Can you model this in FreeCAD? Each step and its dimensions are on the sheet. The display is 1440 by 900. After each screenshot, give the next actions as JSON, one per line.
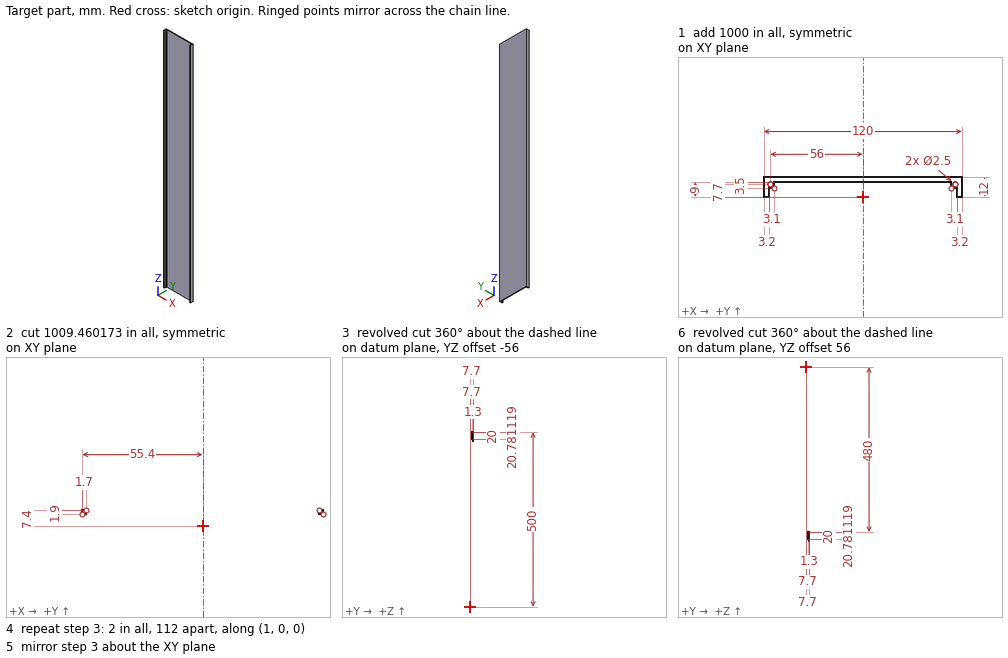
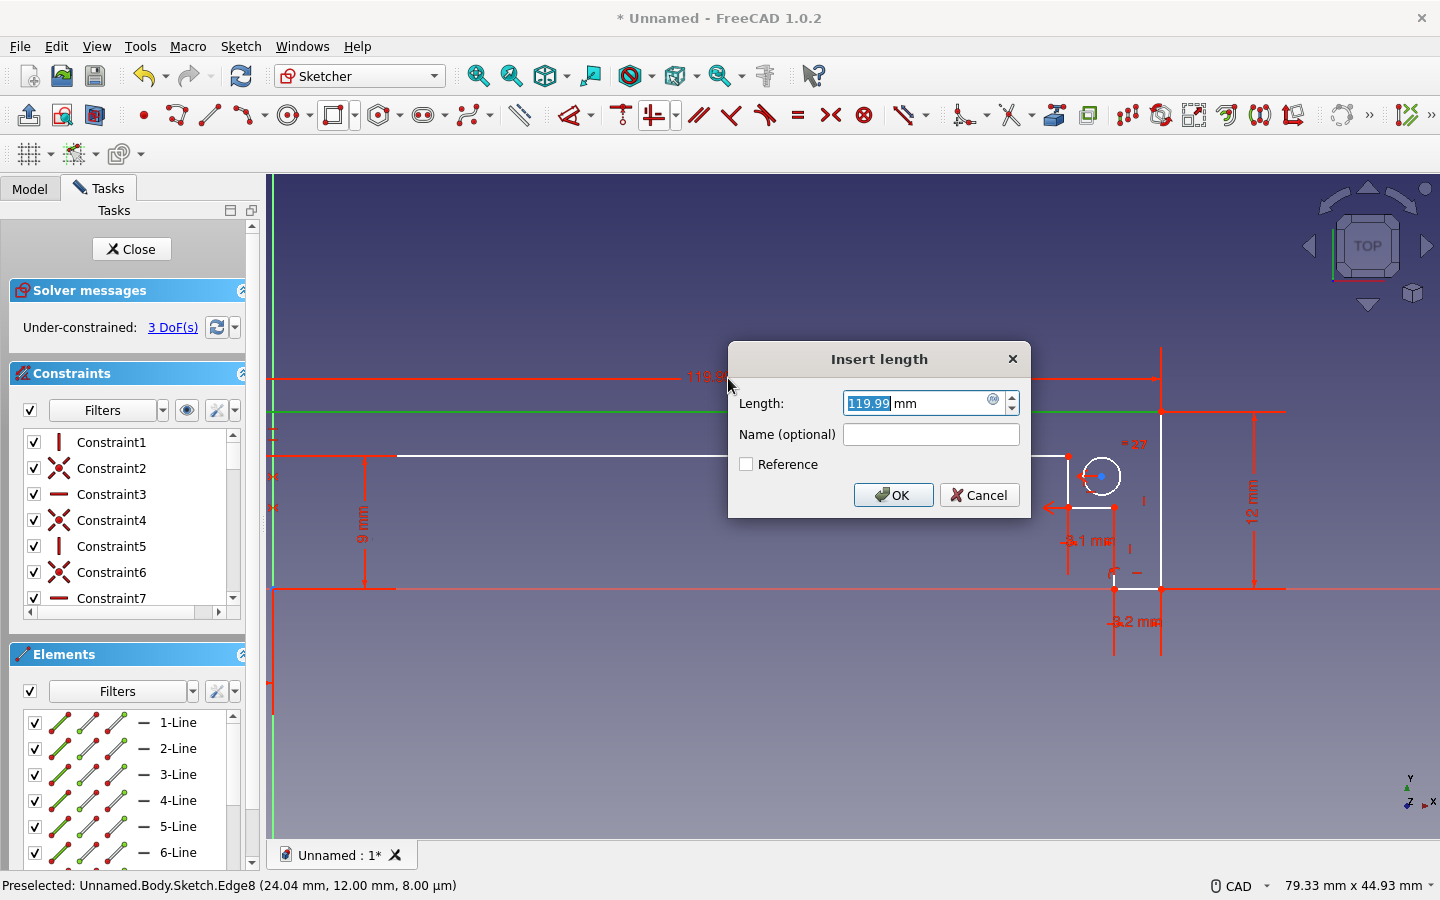
{"action": "type", "text": "120"}
{"action": "key", "text": "Return"}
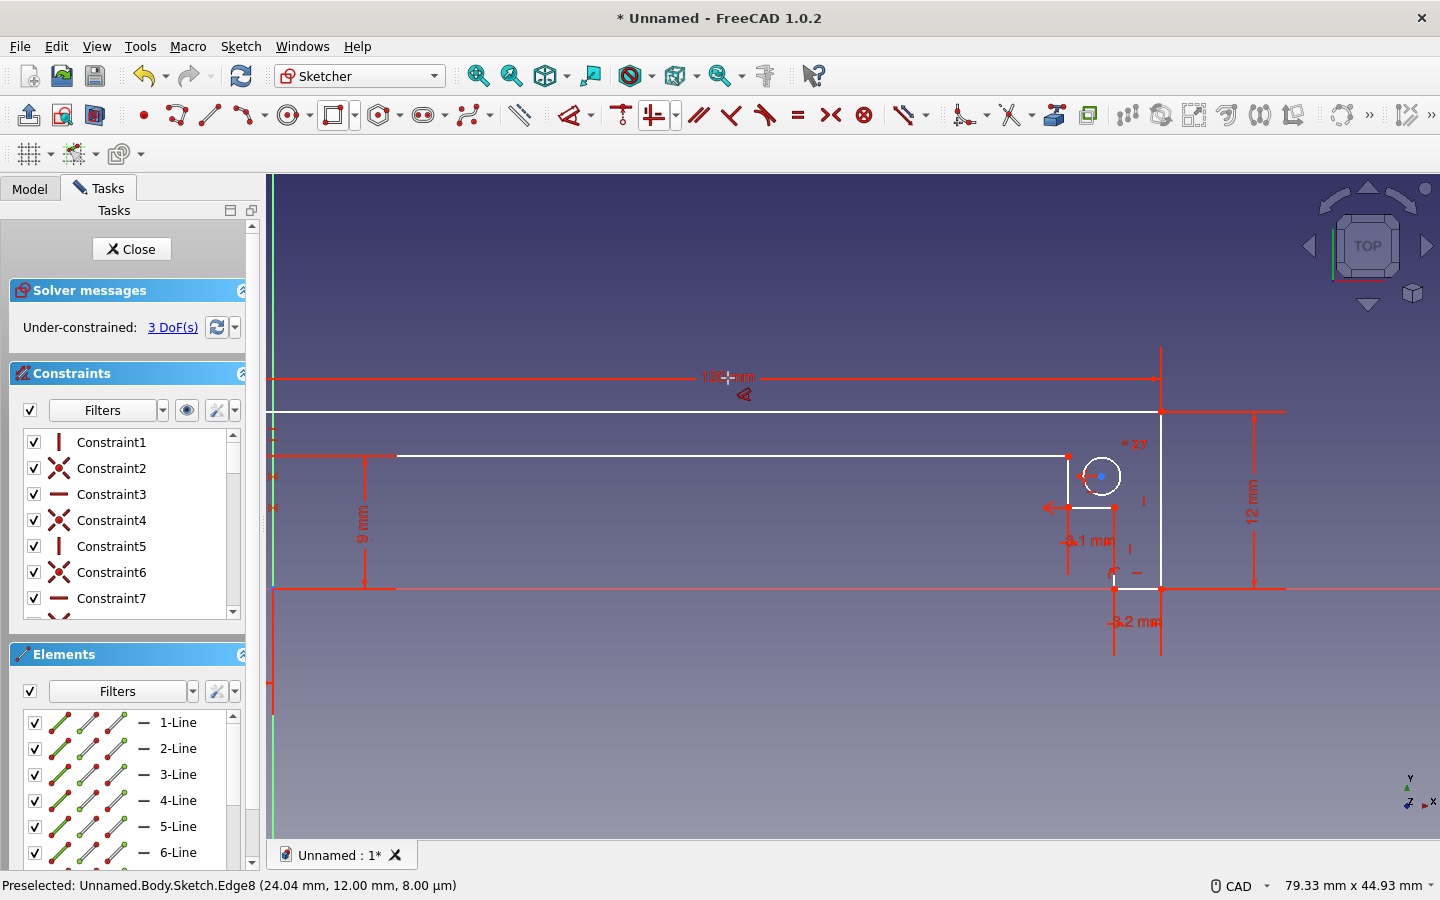
{"action": "scroll", "coordinate": [1082, 510], "scroll_direction": "down", "scroll_amount": 5}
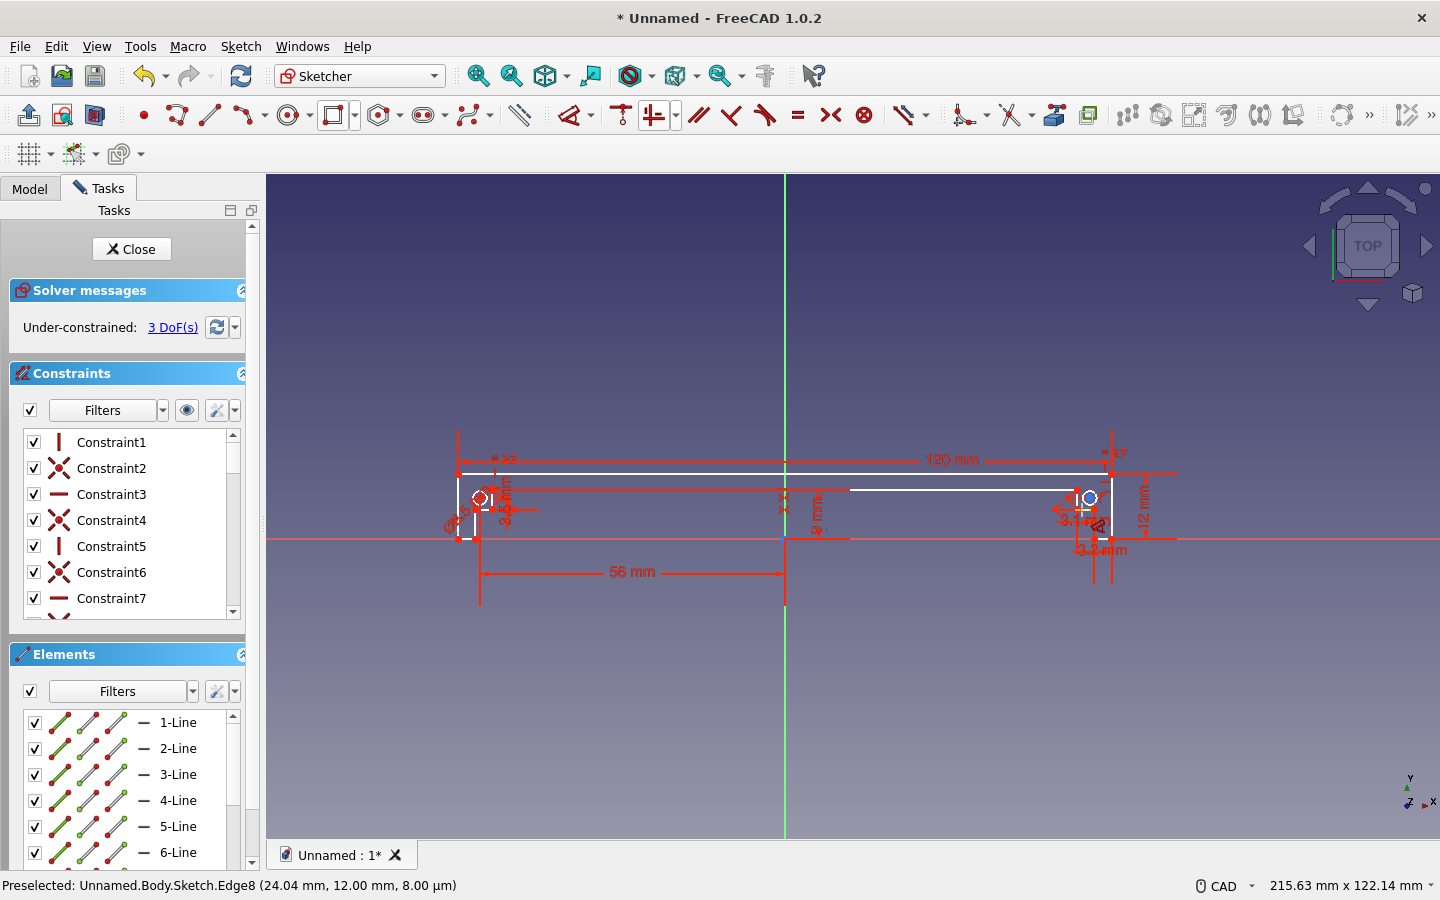
{"action": "scroll", "coordinate": [463, 539], "scroll_direction": "up", "scroll_amount": 5}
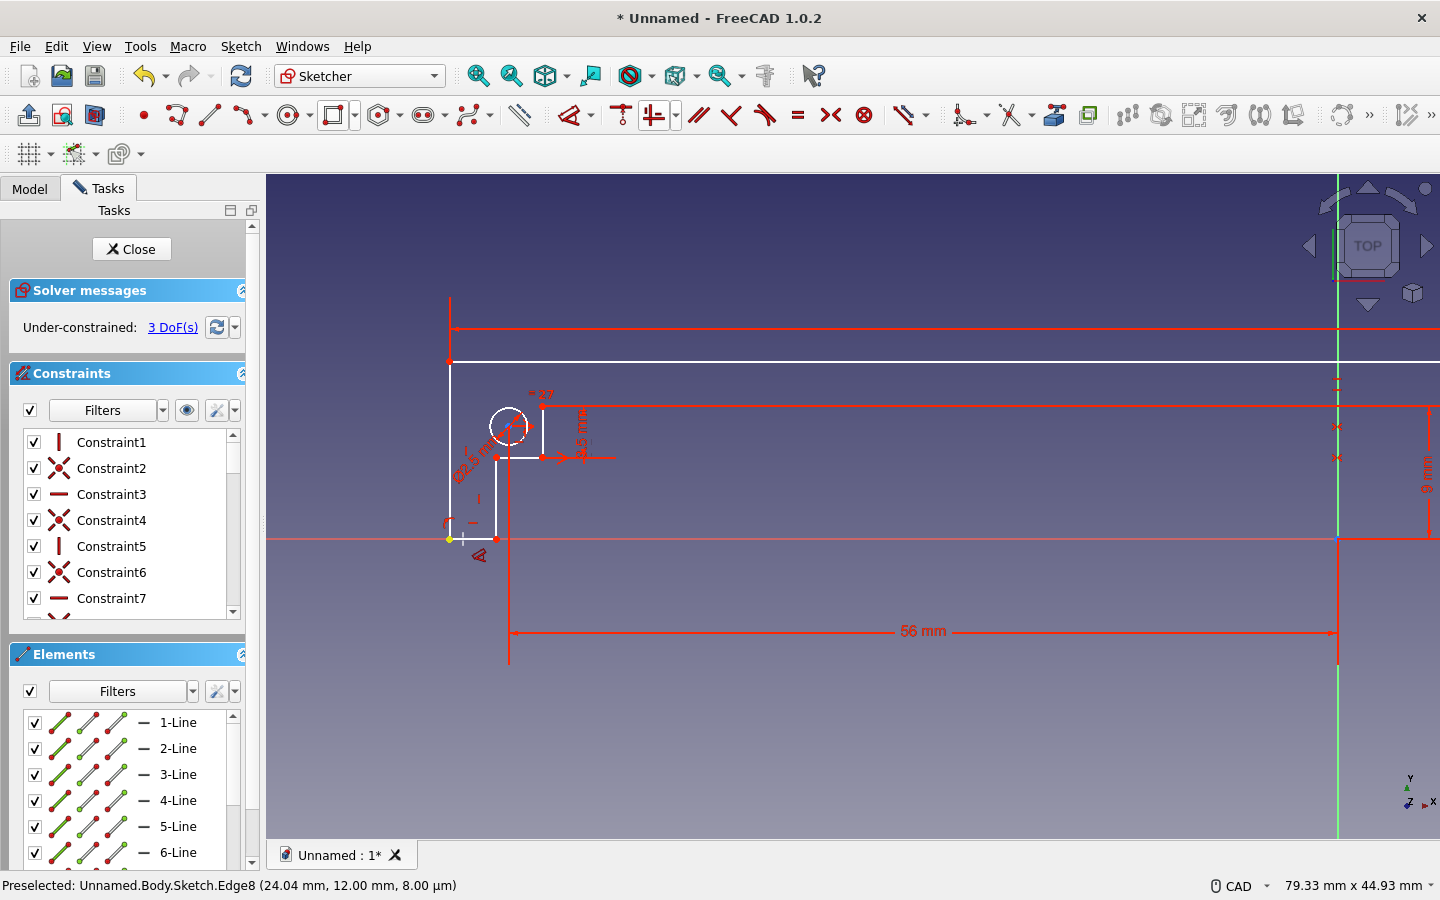
{"action": "left_click", "coordinate": [464, 539]}
{"action": "left_click", "coordinate": [473, 573]}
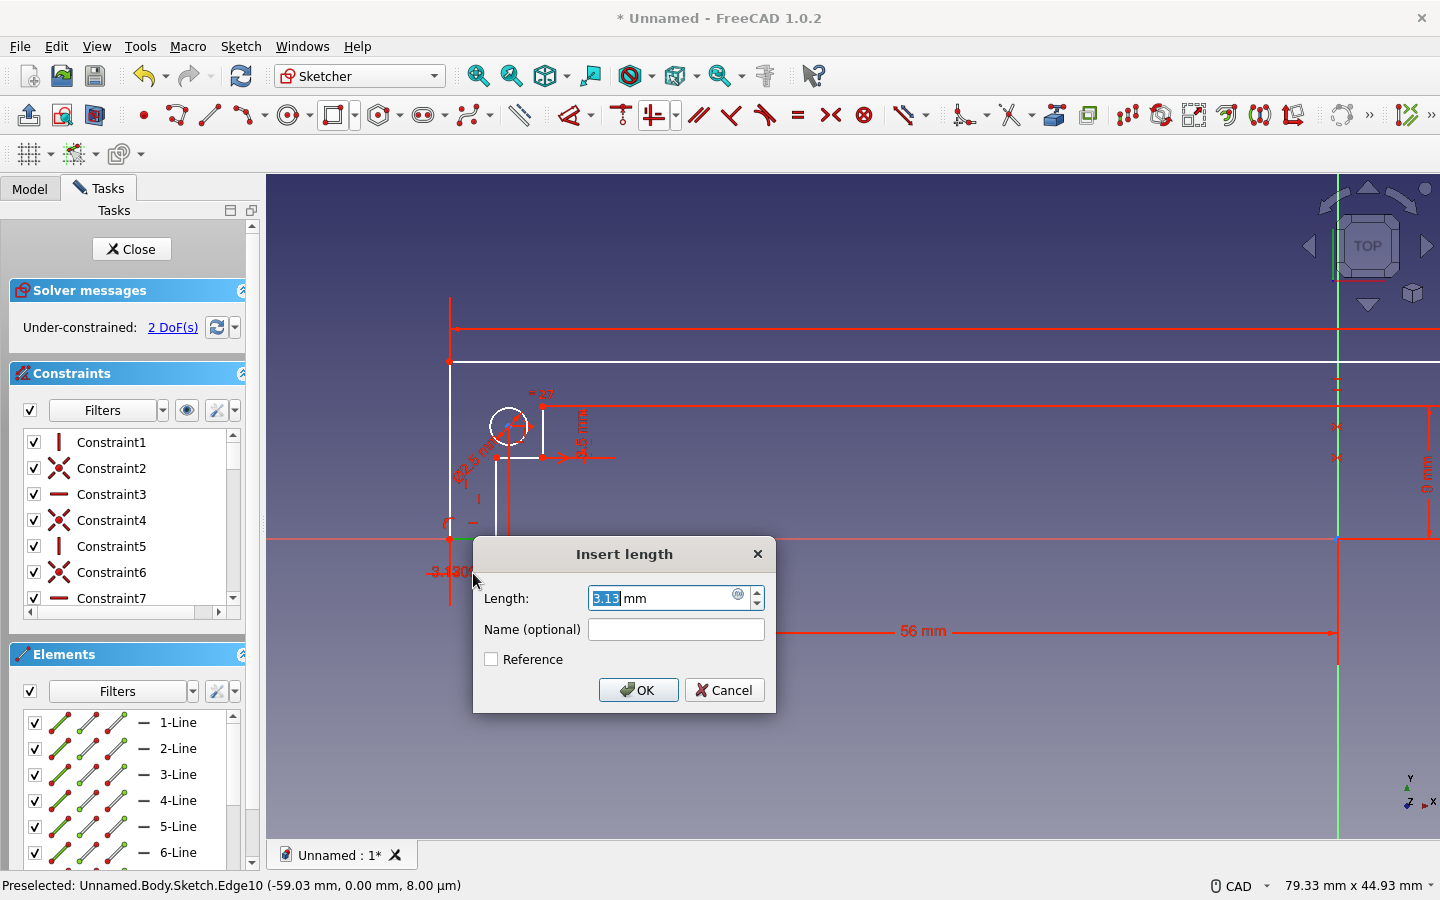
{"action": "type", "text": "3.2"}
{"action": "key", "text": "Return"}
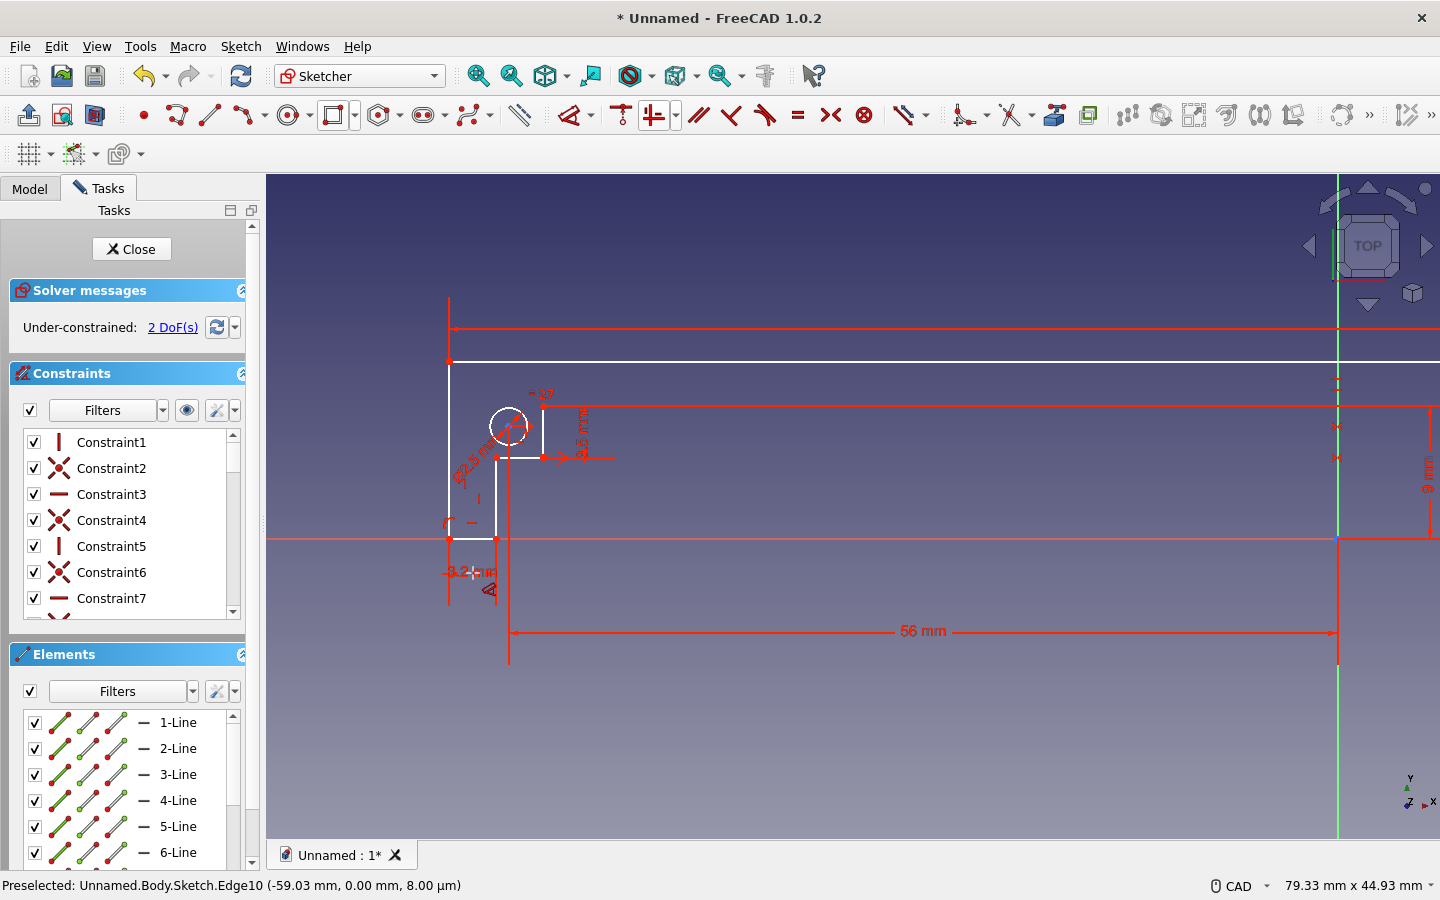
{"action": "left_click", "coordinate": [511, 458]}
{"action": "left_click", "coordinate": [520, 492]}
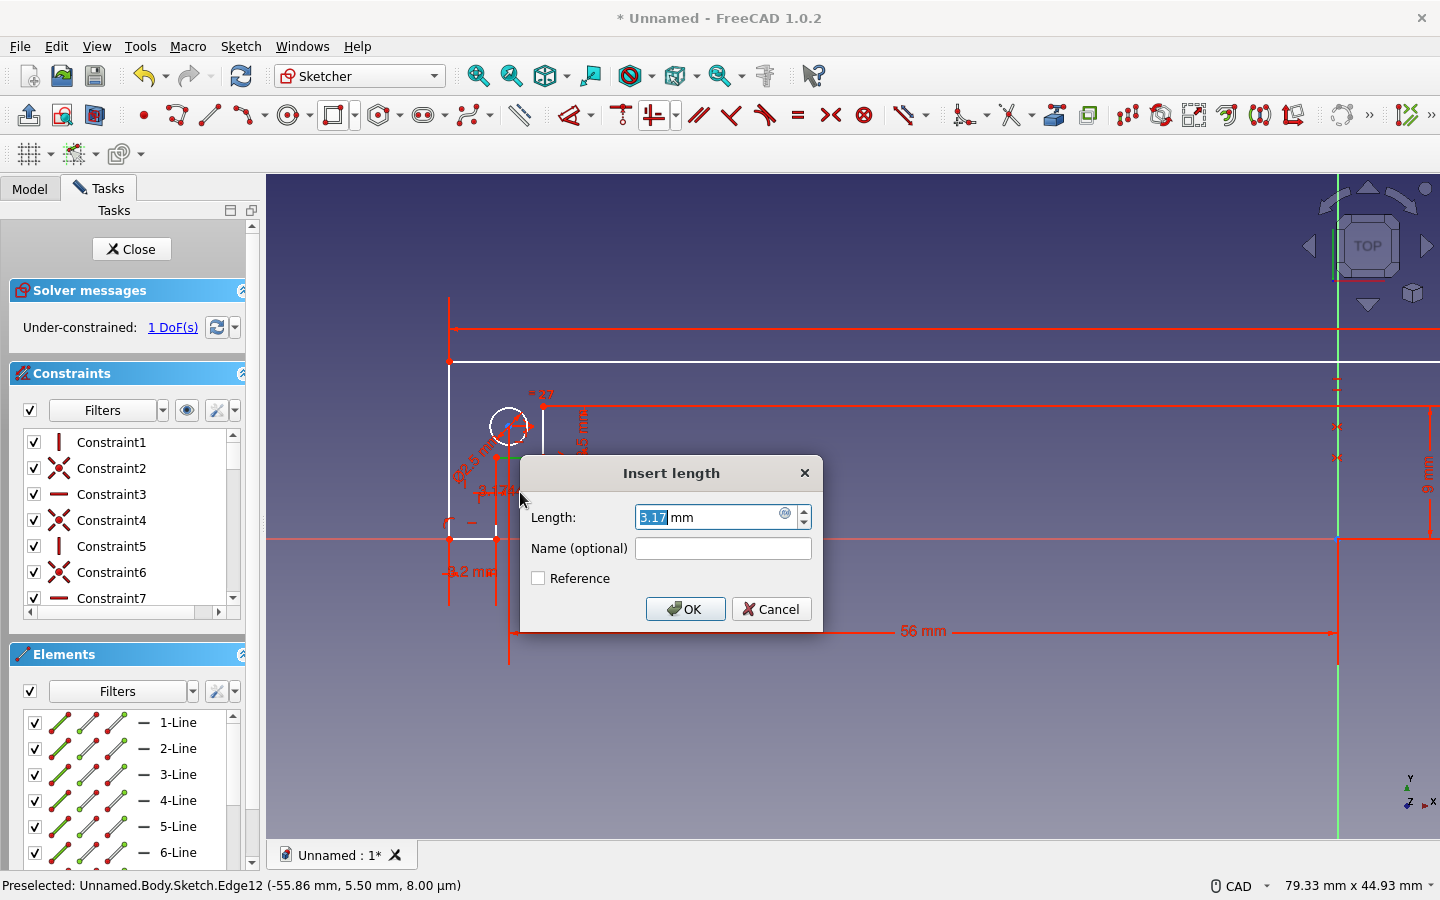
{"action": "type", "text": "3.1"}
{"action": "key", "text": "Return"}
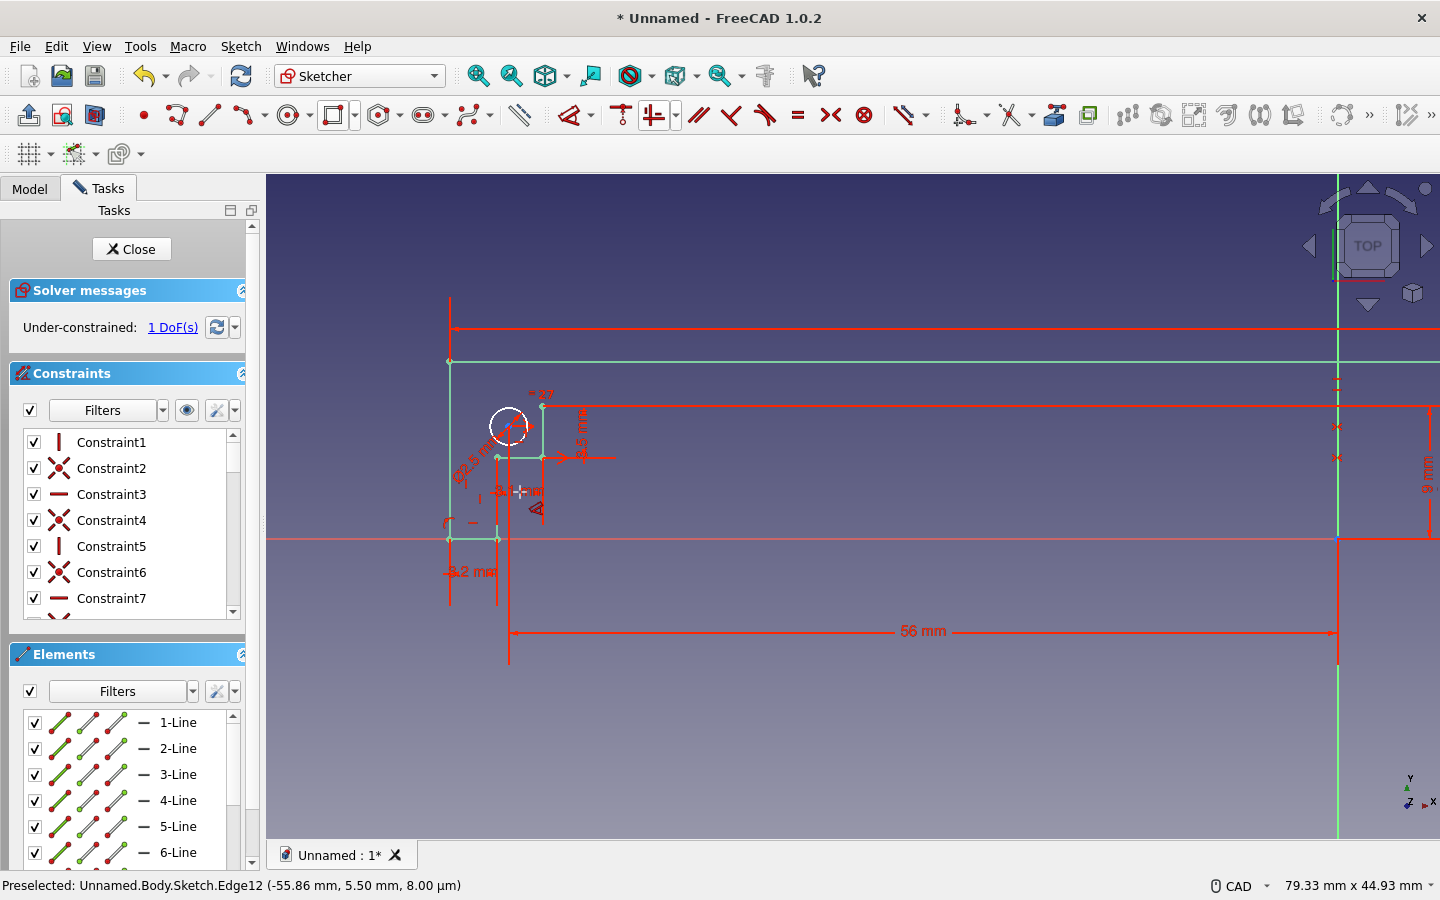
{"action": "left_click", "coordinate": [509, 426]}
{"action": "left_click", "coordinate": [475, 522]}